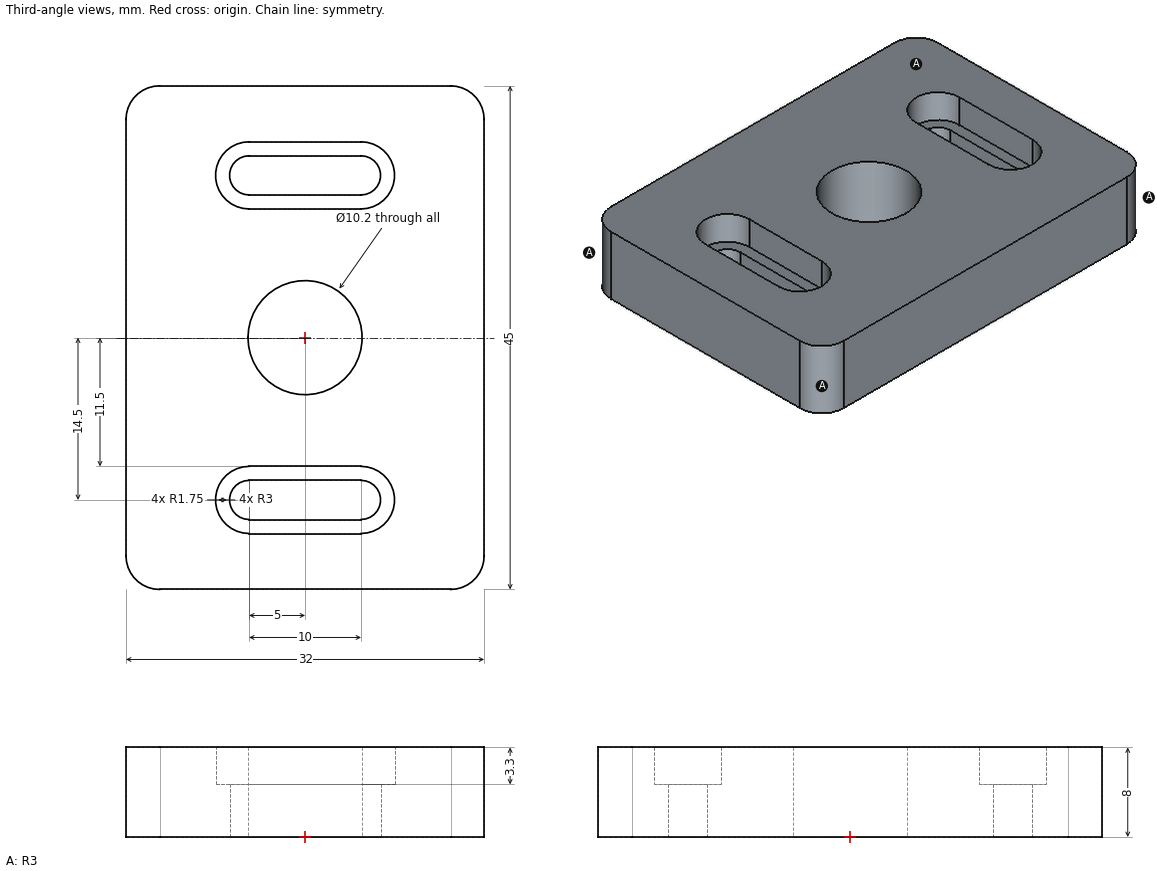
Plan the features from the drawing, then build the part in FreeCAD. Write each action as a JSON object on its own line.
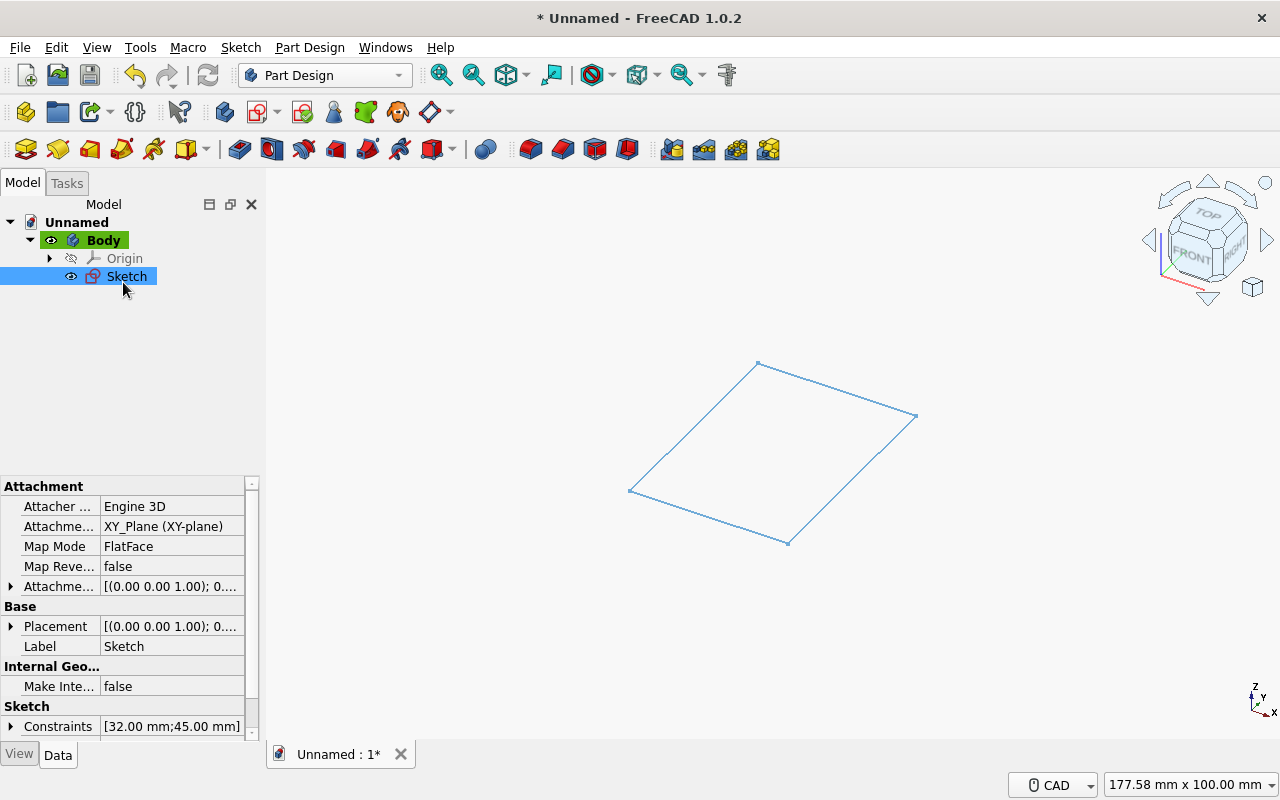
{"action": "left_click", "coordinate": [26, 150]}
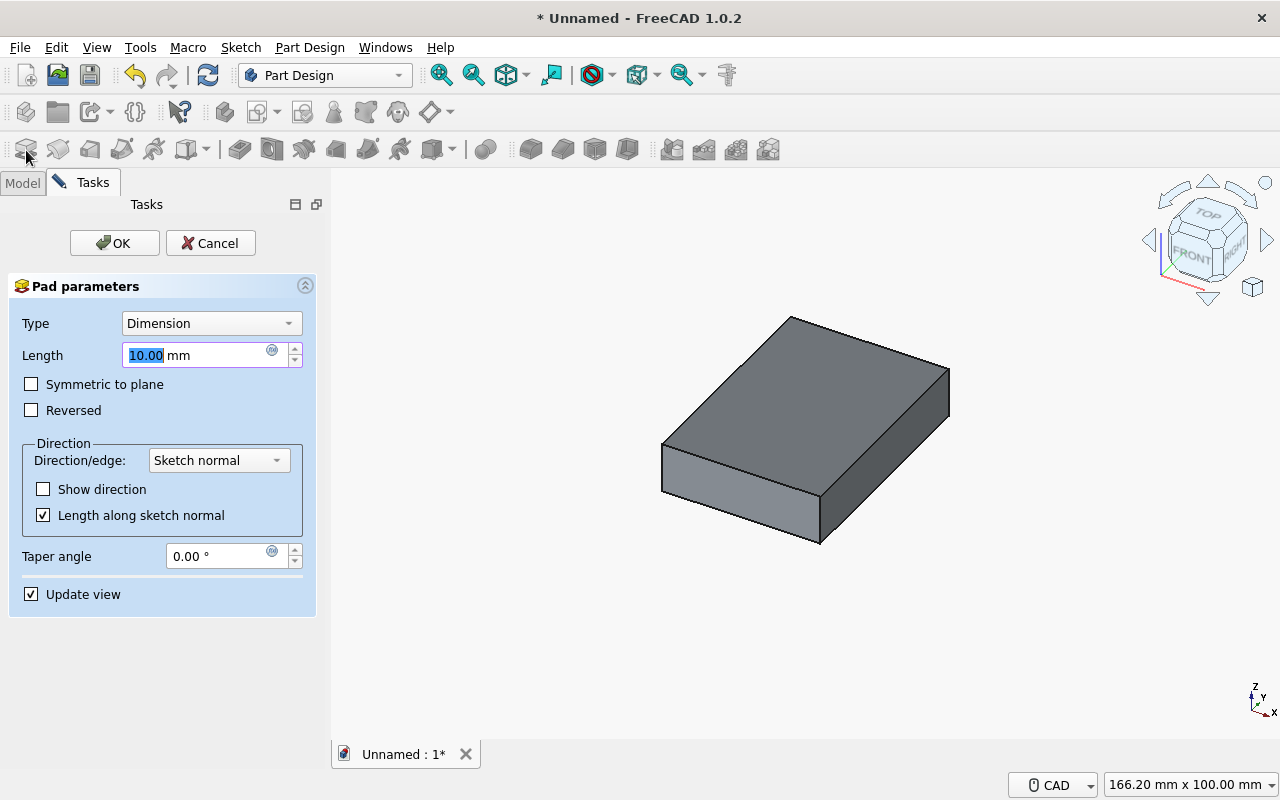
{"action": "type", "text": "8"}
{"action": "key", "text": "Tab"}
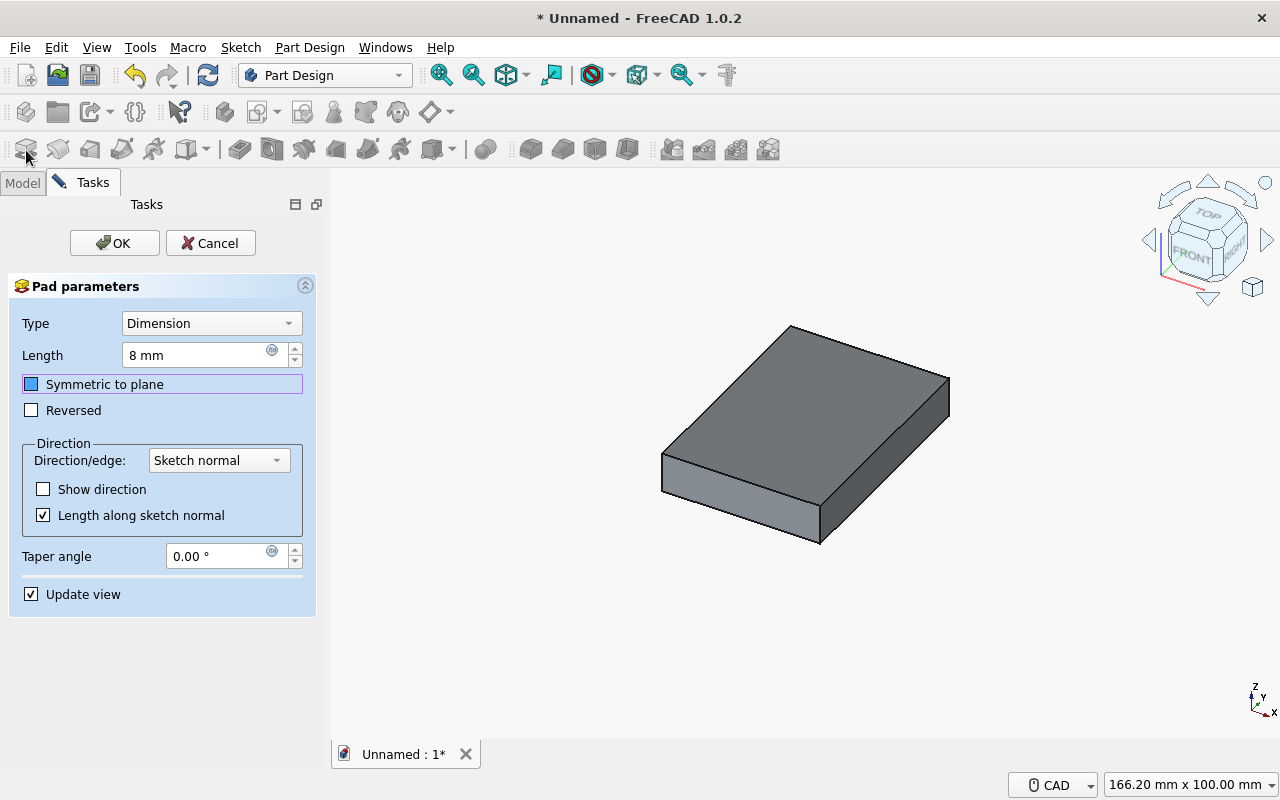
{"action": "left_click", "coordinate": [115, 243]}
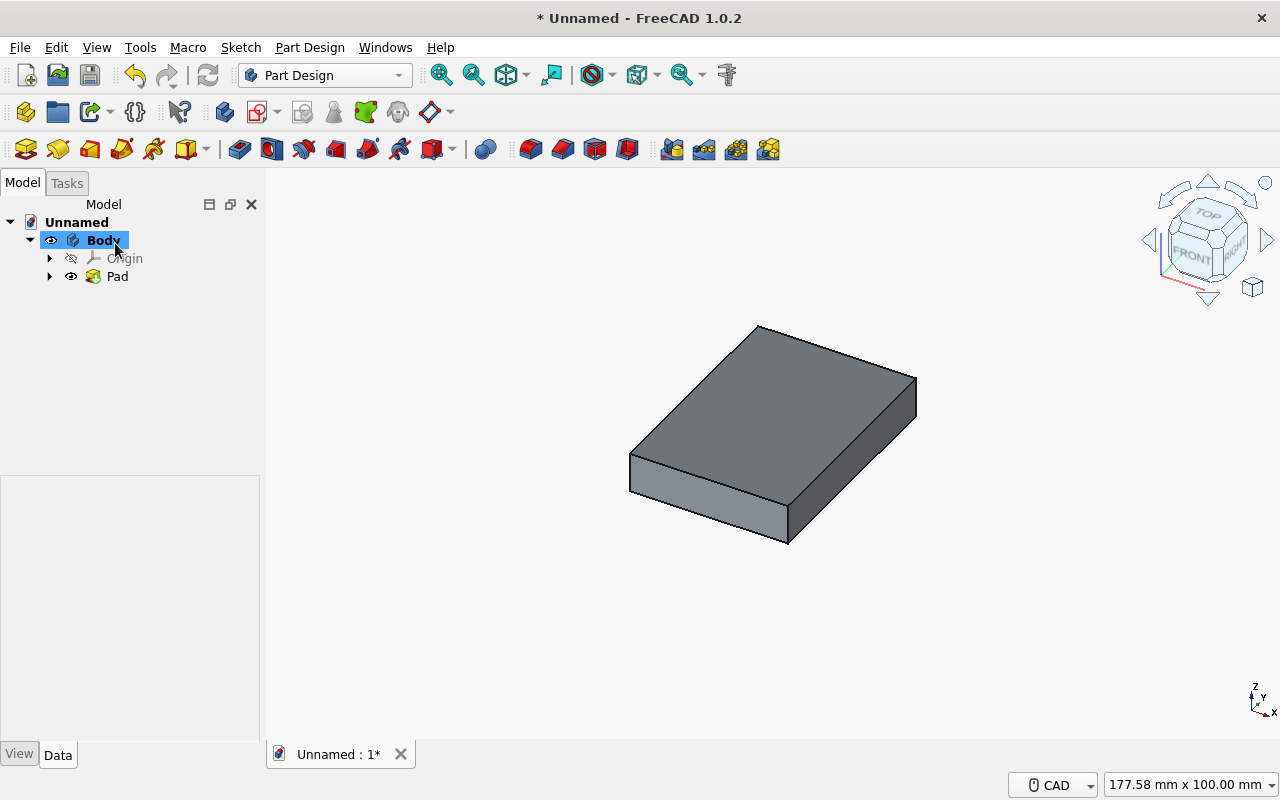
{"action": "left_click", "coordinate": [442, 76]}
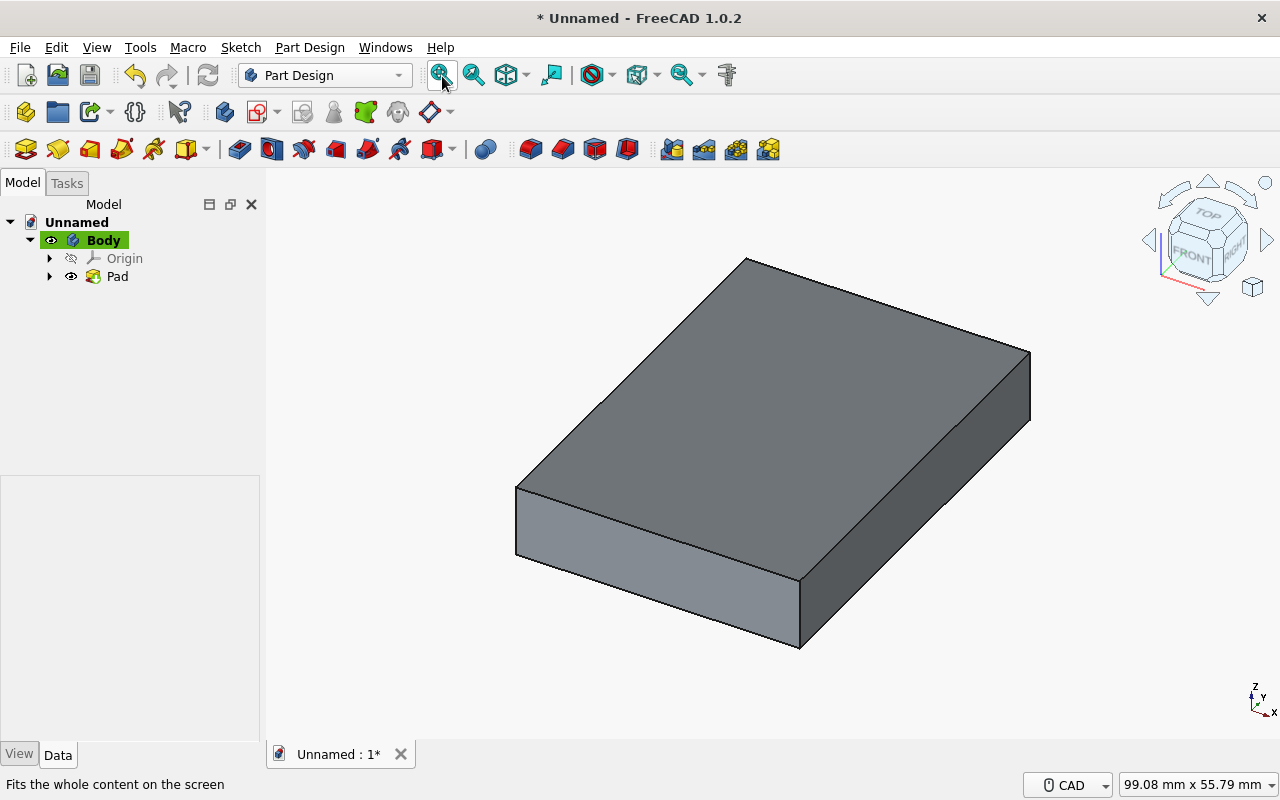
{"action": "left_click", "coordinate": [806, 386]}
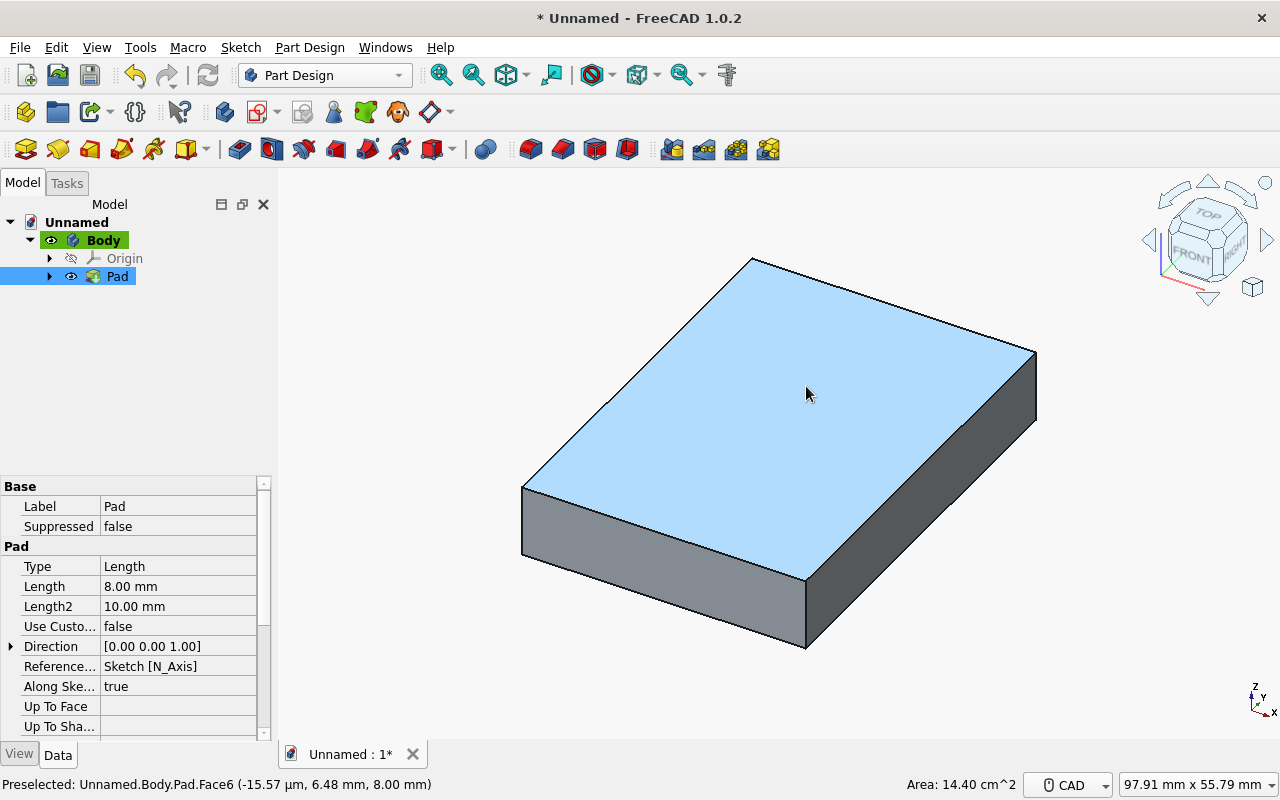
{"action": "left_click", "coordinate": [258, 112]}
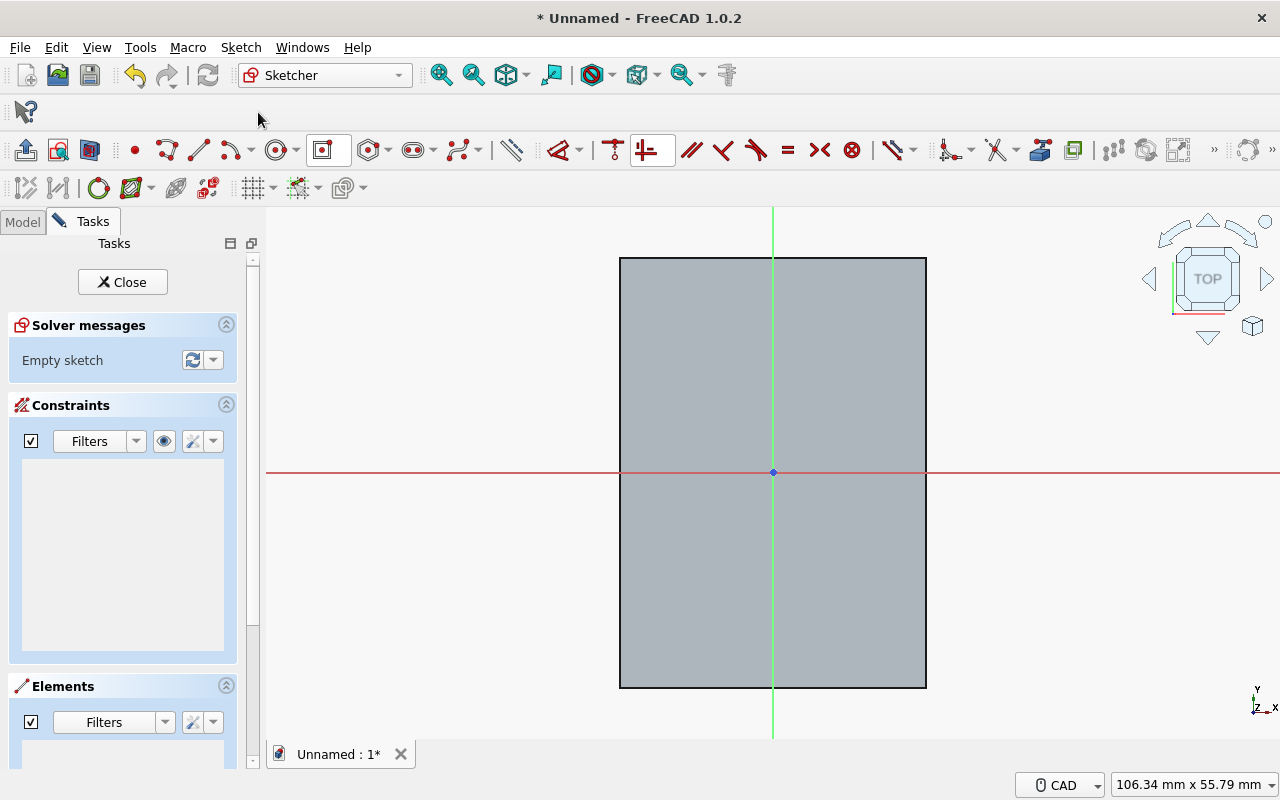
{"action": "scroll", "coordinate": [803, 473], "scroll_direction": "up", "scroll_amount": 6}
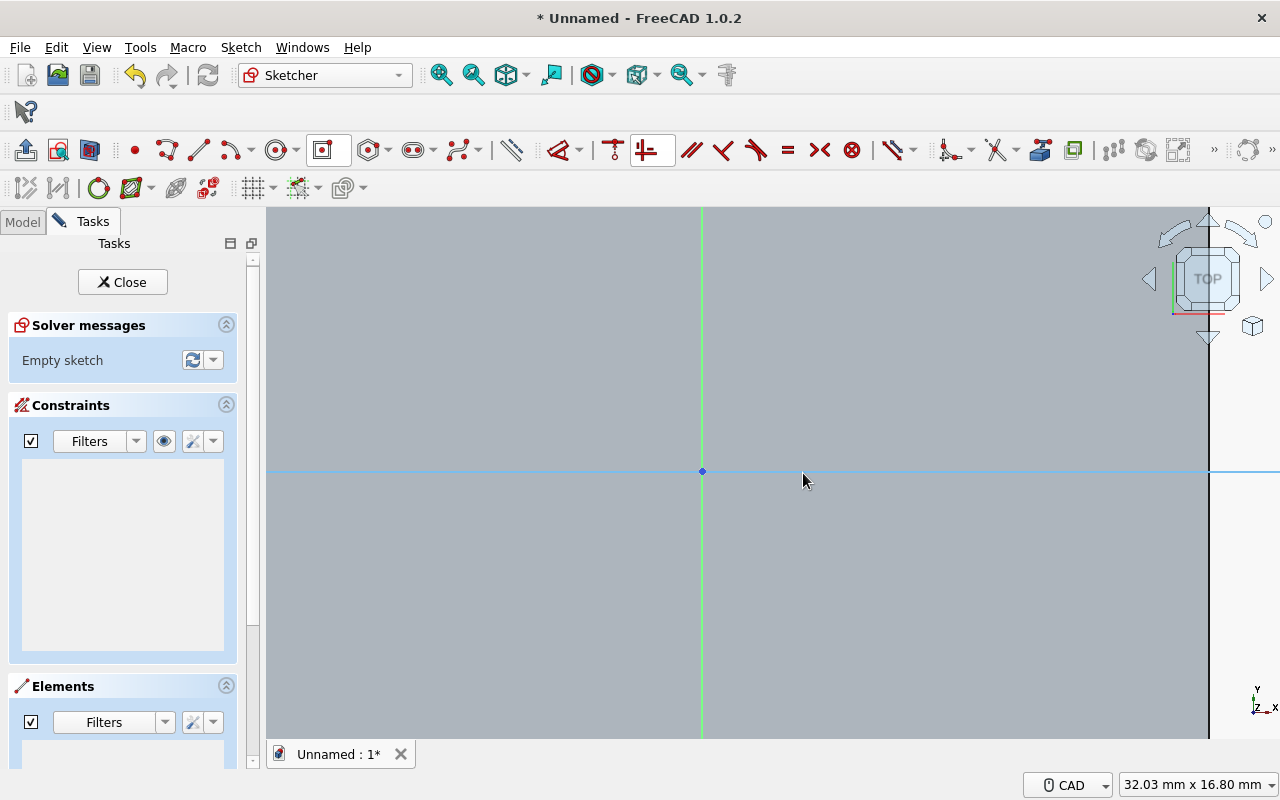
{"action": "left_click", "coordinate": [276, 150]}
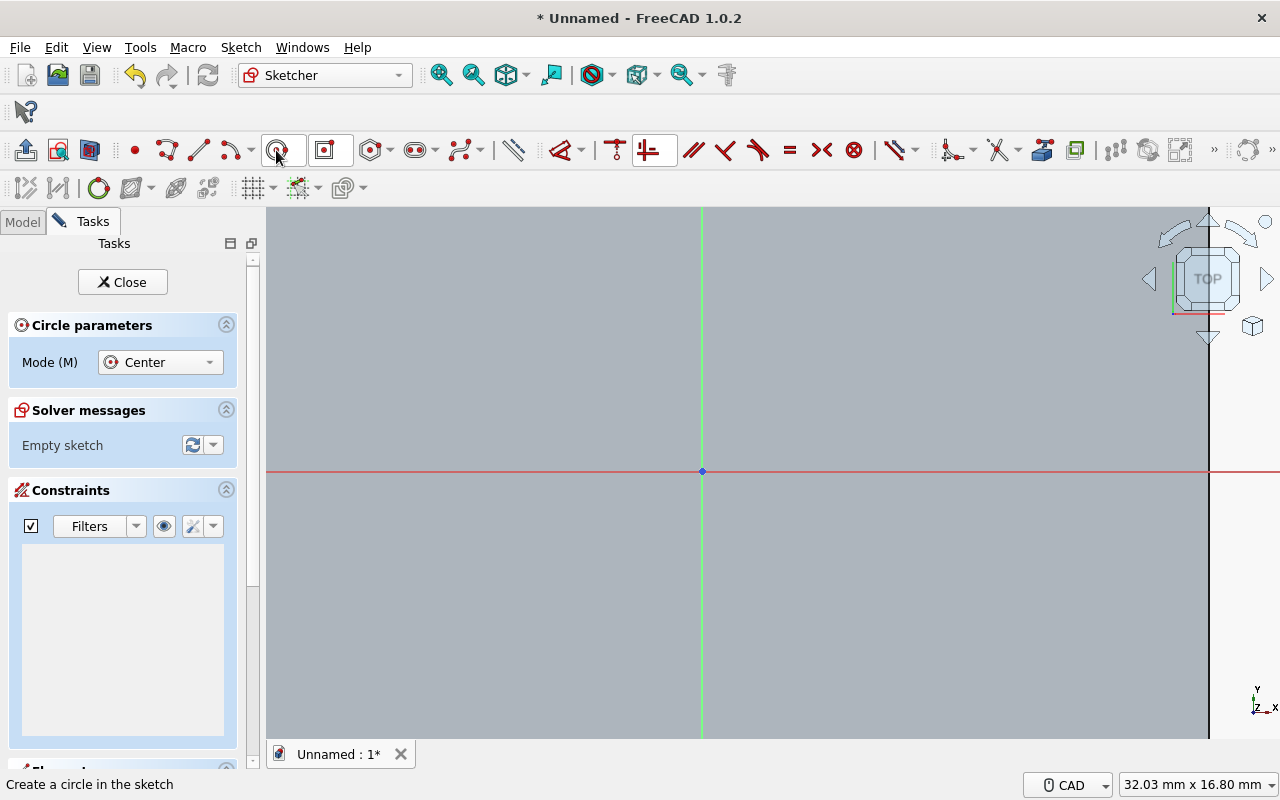
{"action": "left_click", "coordinate": [702, 472]}
{"action": "mouse_move", "coordinate": [816, 358]}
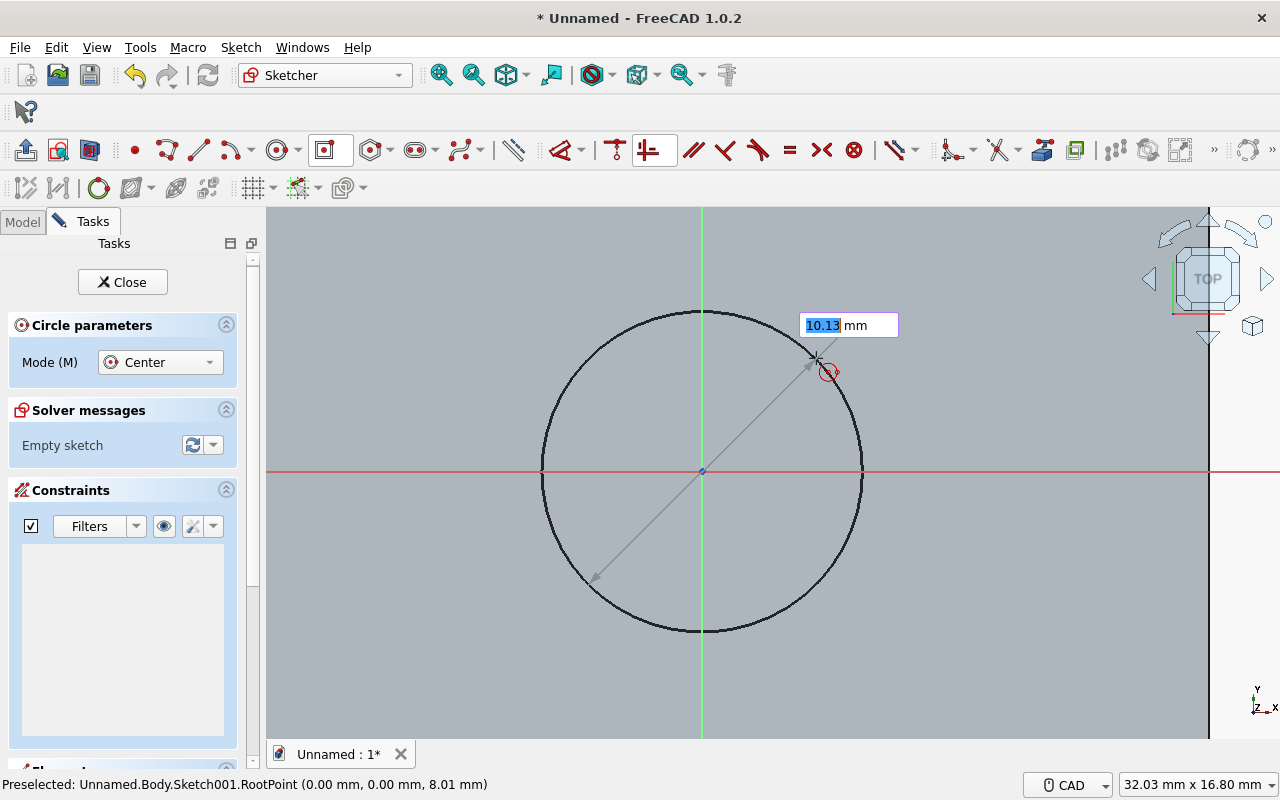
{"action": "type", "text": "10.2"}
{"action": "key", "text": "Return"}
{"action": "key", "text": "Escape"}